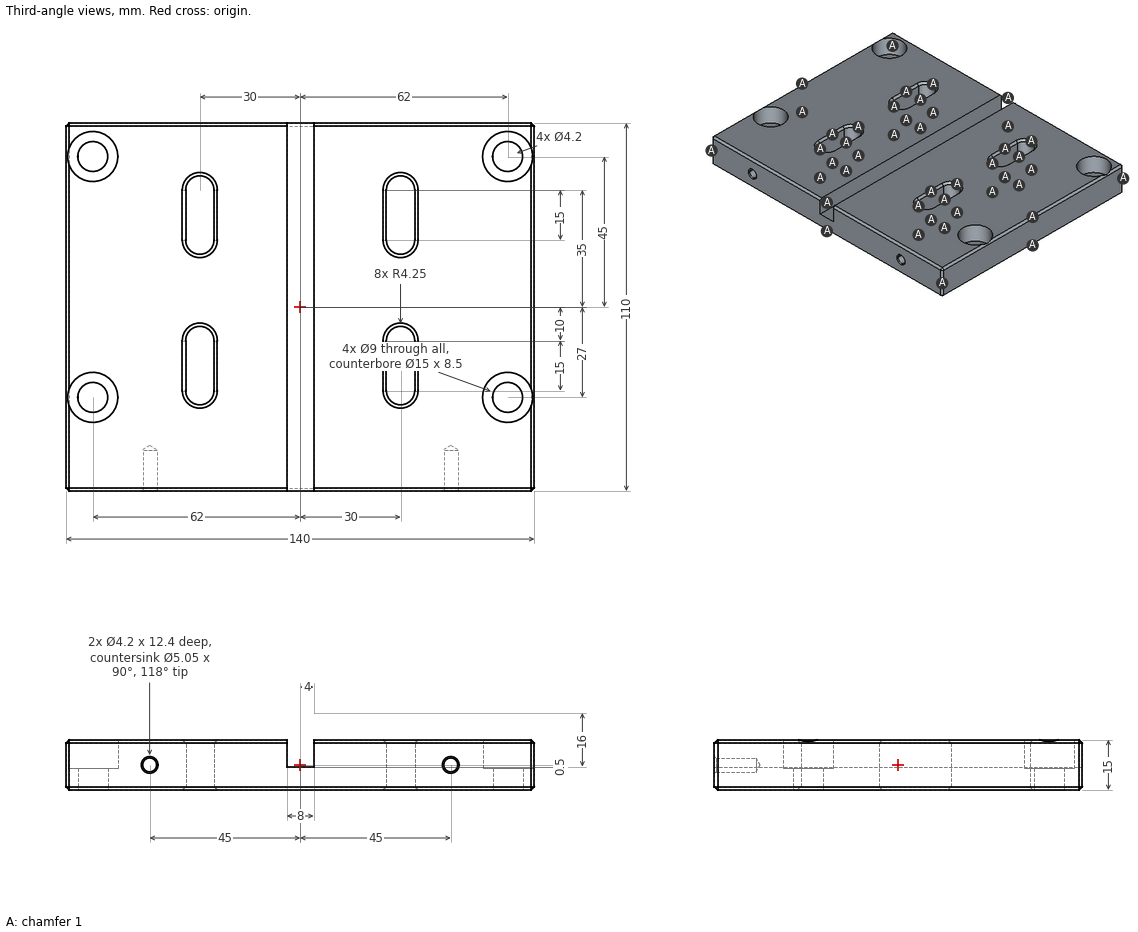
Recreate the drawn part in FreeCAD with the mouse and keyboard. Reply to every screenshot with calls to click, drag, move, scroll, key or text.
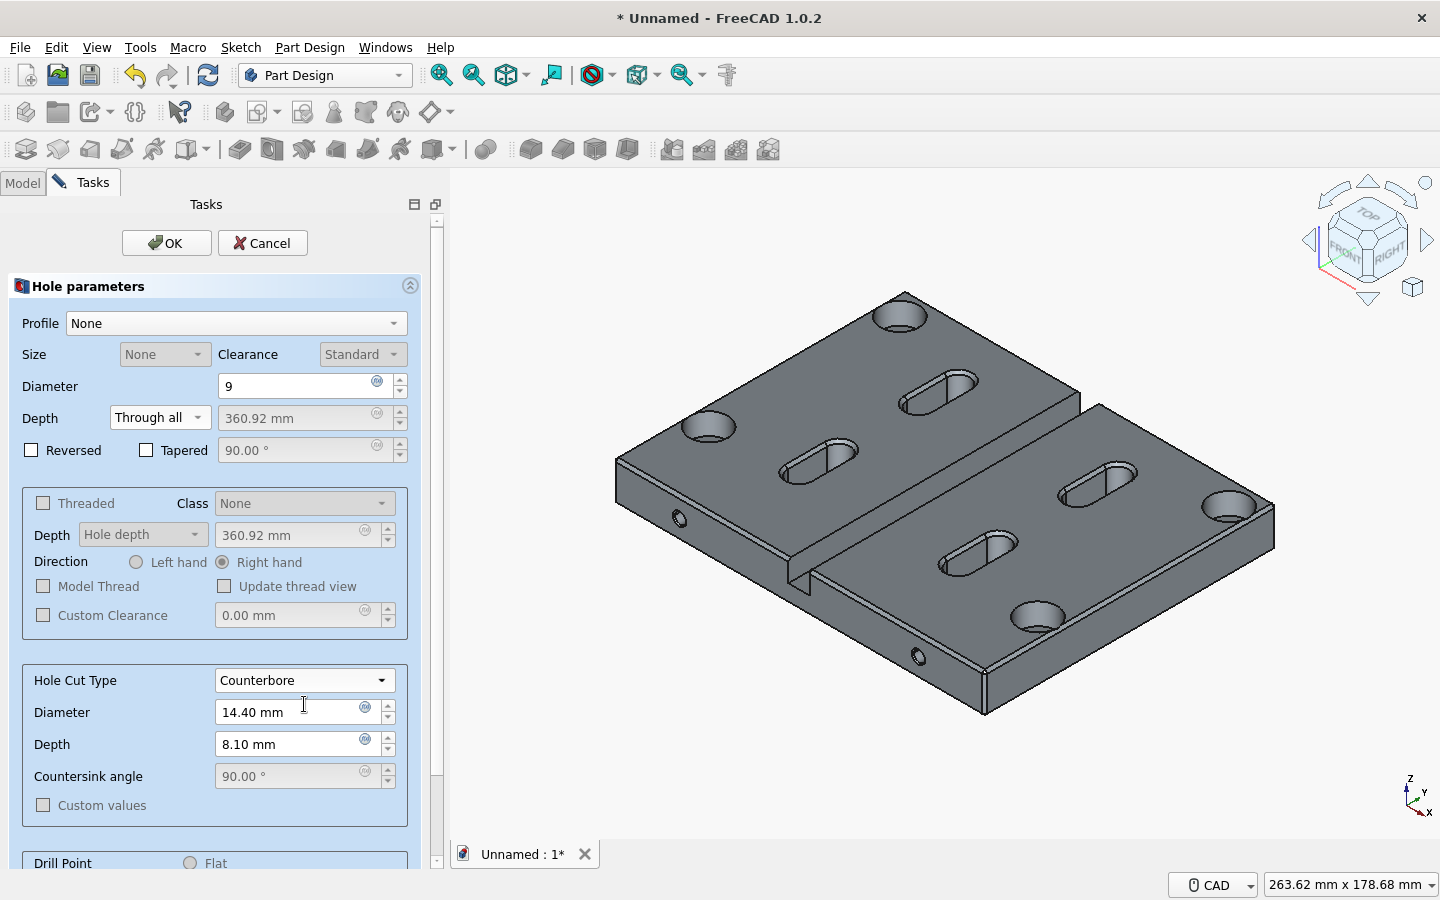
triple_click(298, 712)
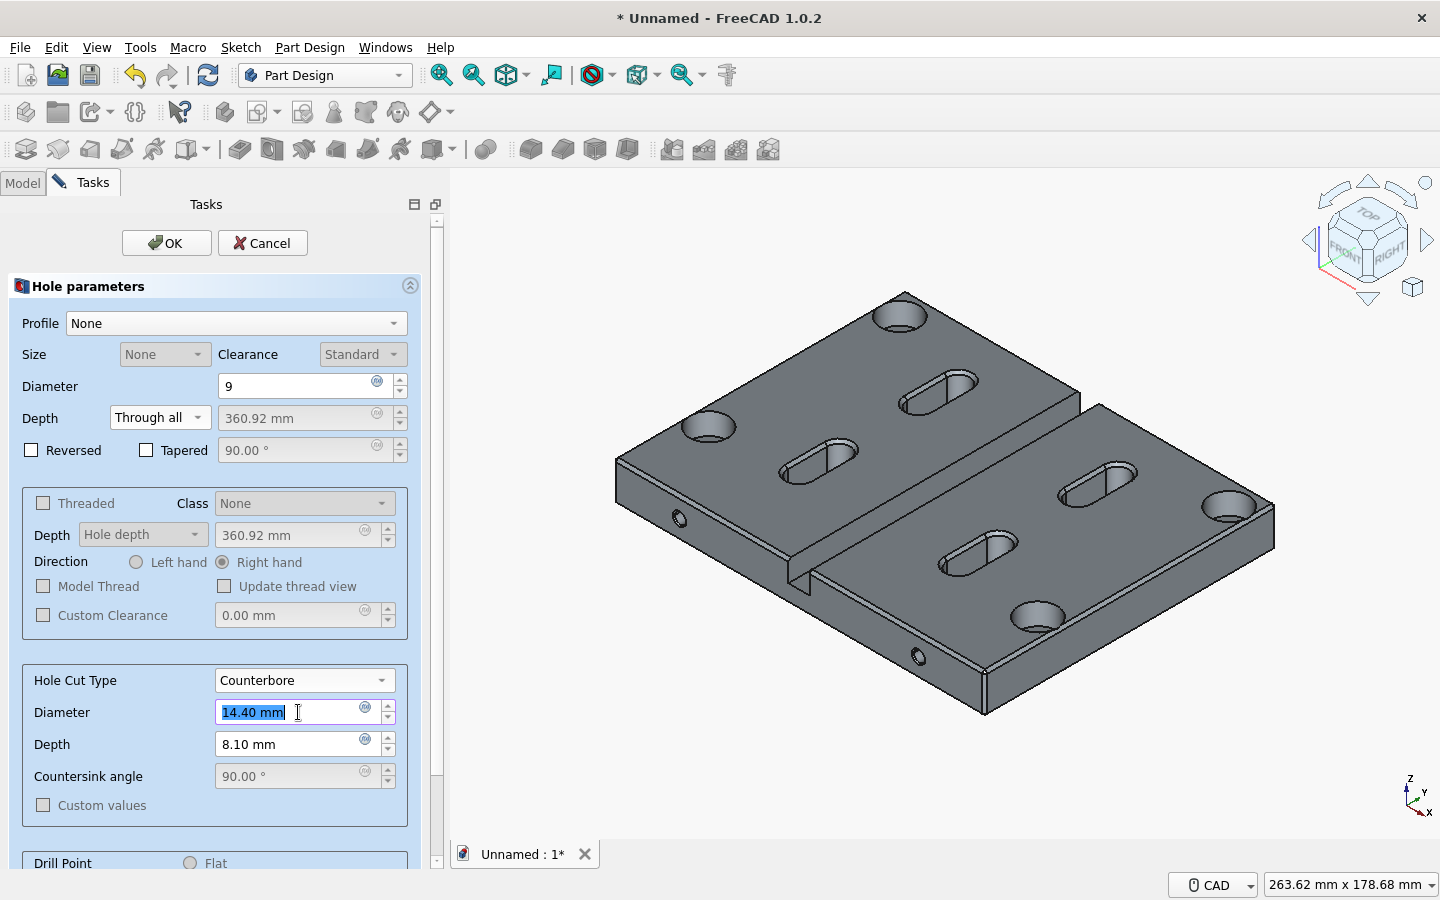
text(15)
key(Tab)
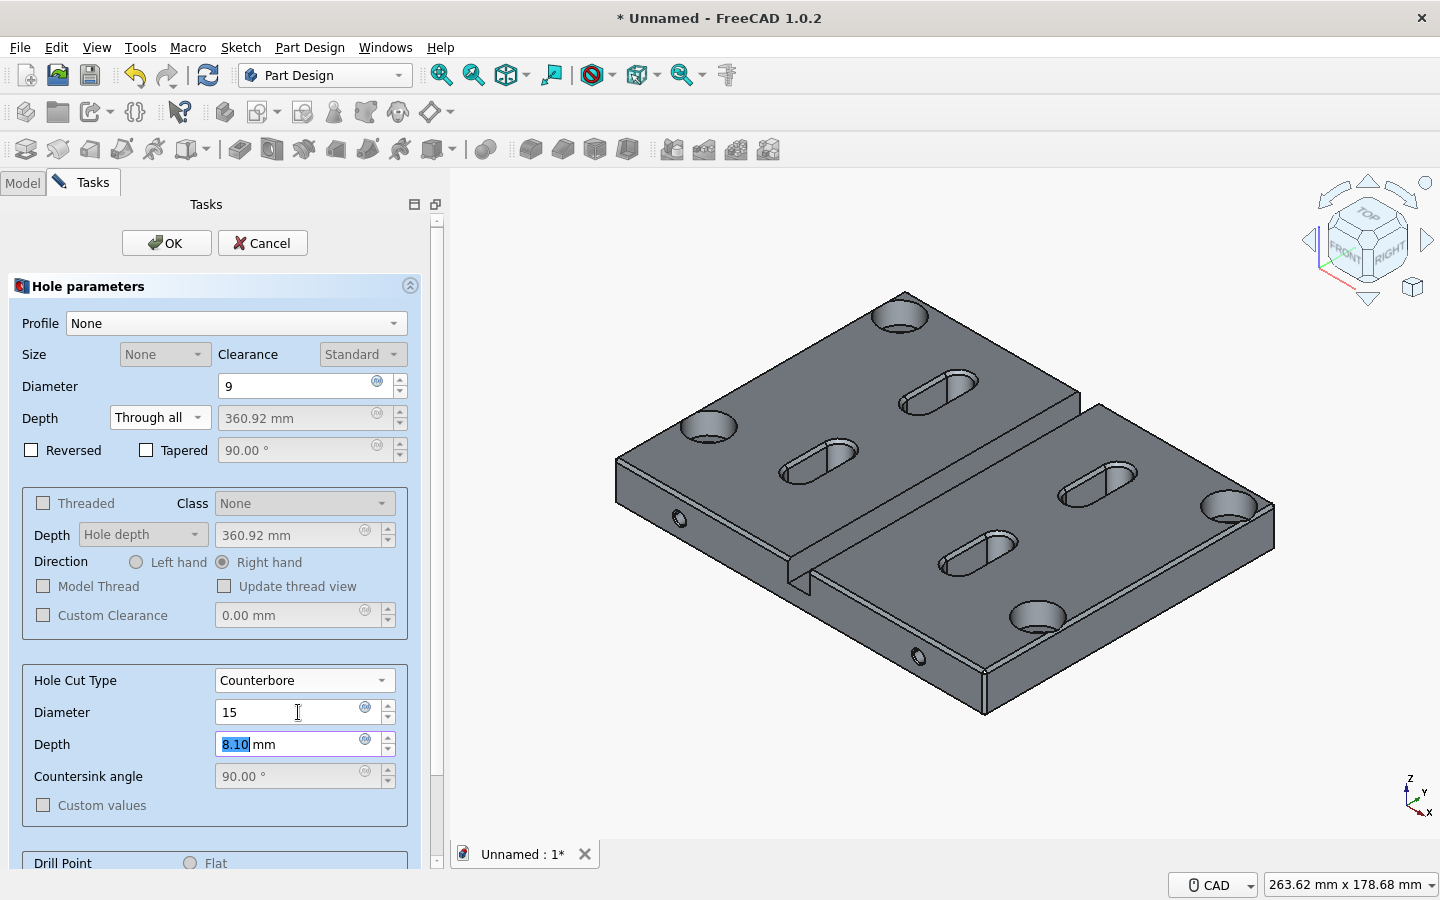
text(8.5)
key(Tab)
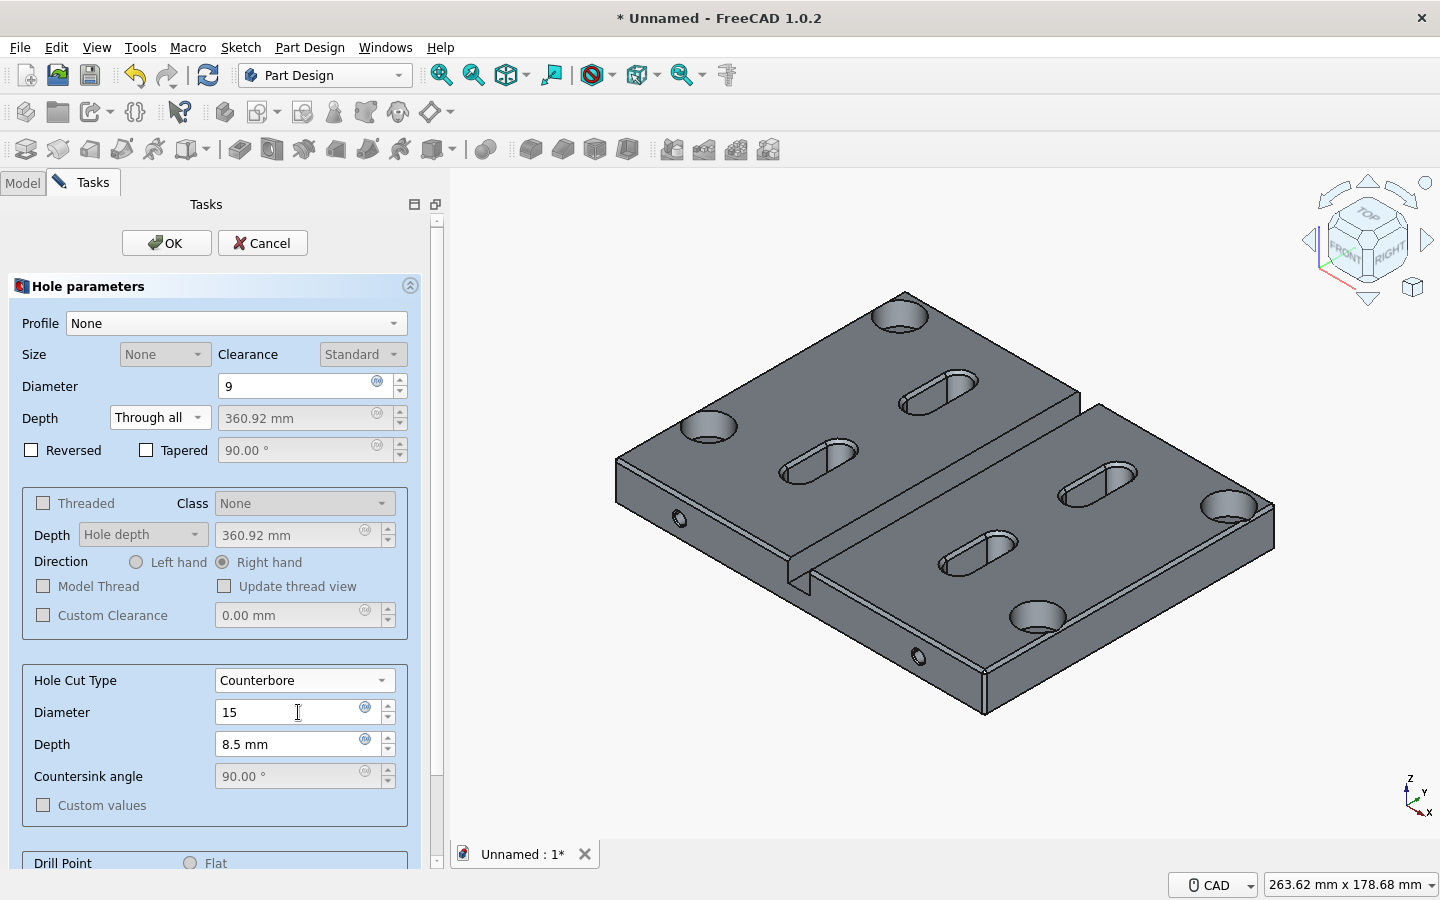
click(167, 243)